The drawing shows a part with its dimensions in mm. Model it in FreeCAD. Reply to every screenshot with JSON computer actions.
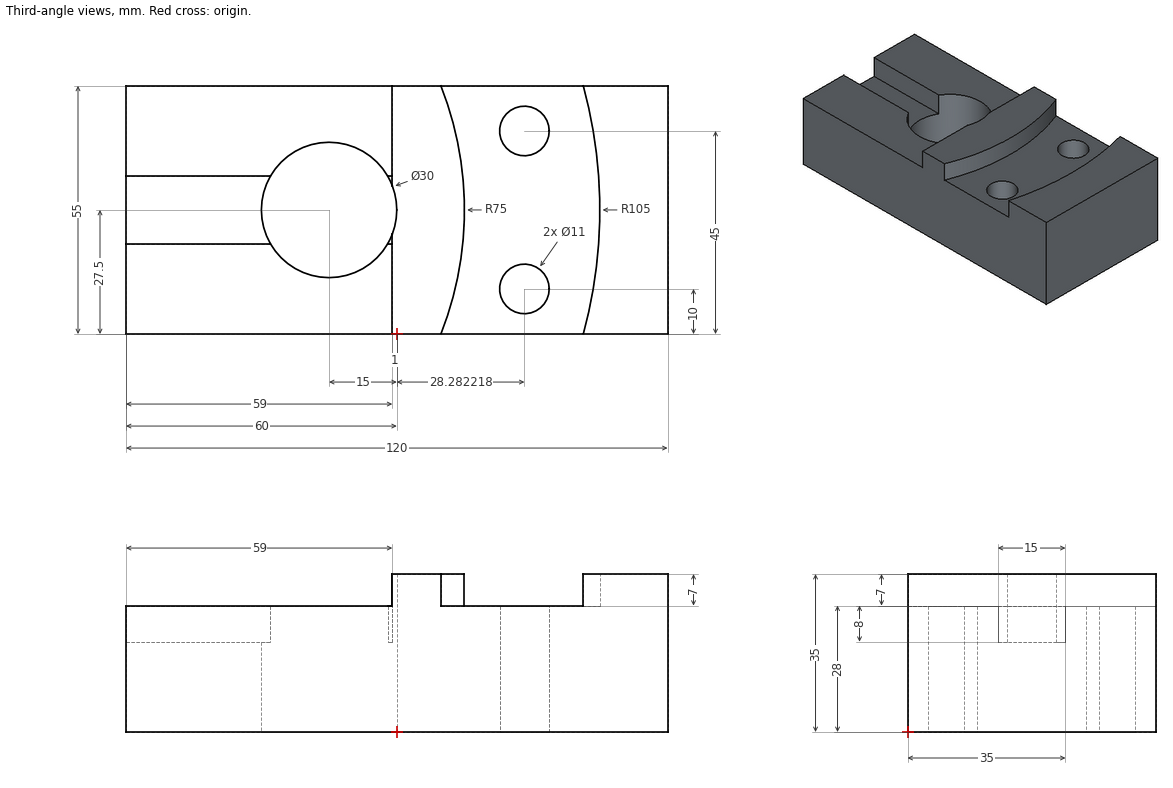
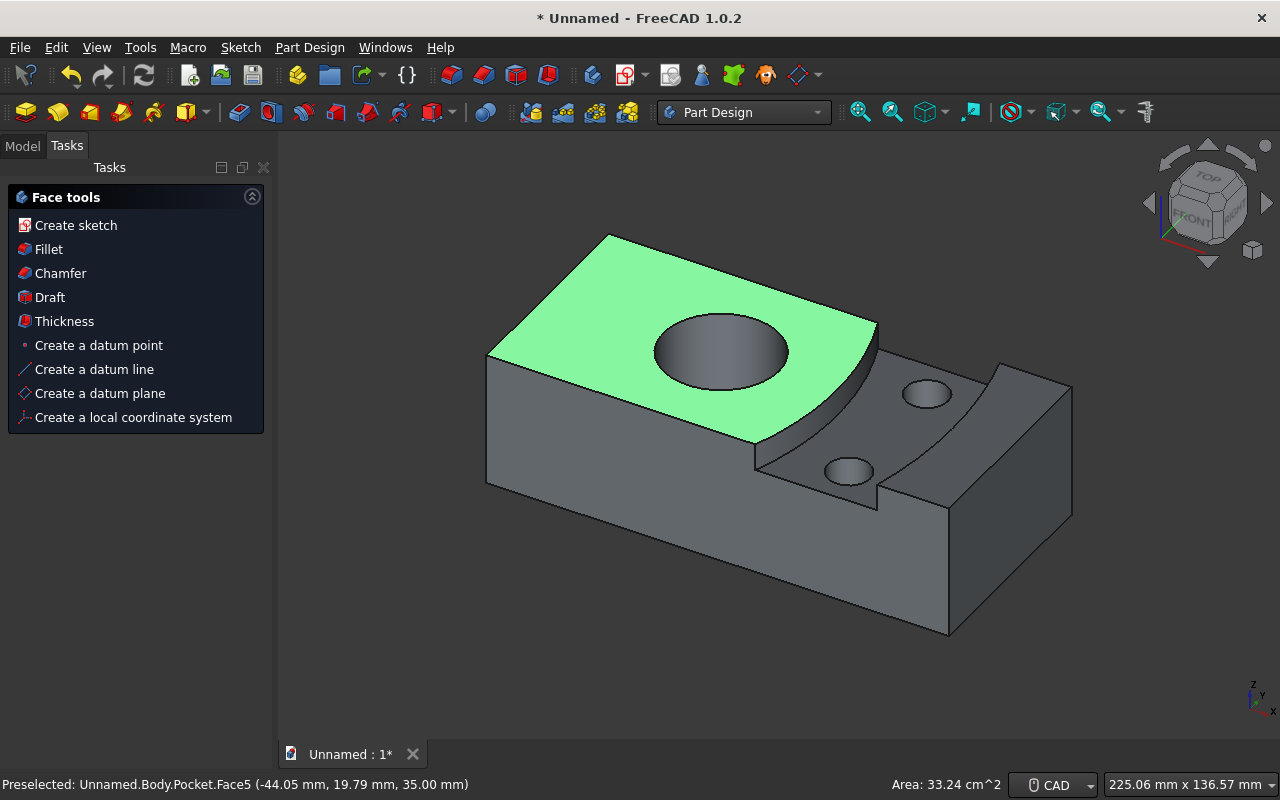
{"action": "left_click", "coordinate": [626, 76]}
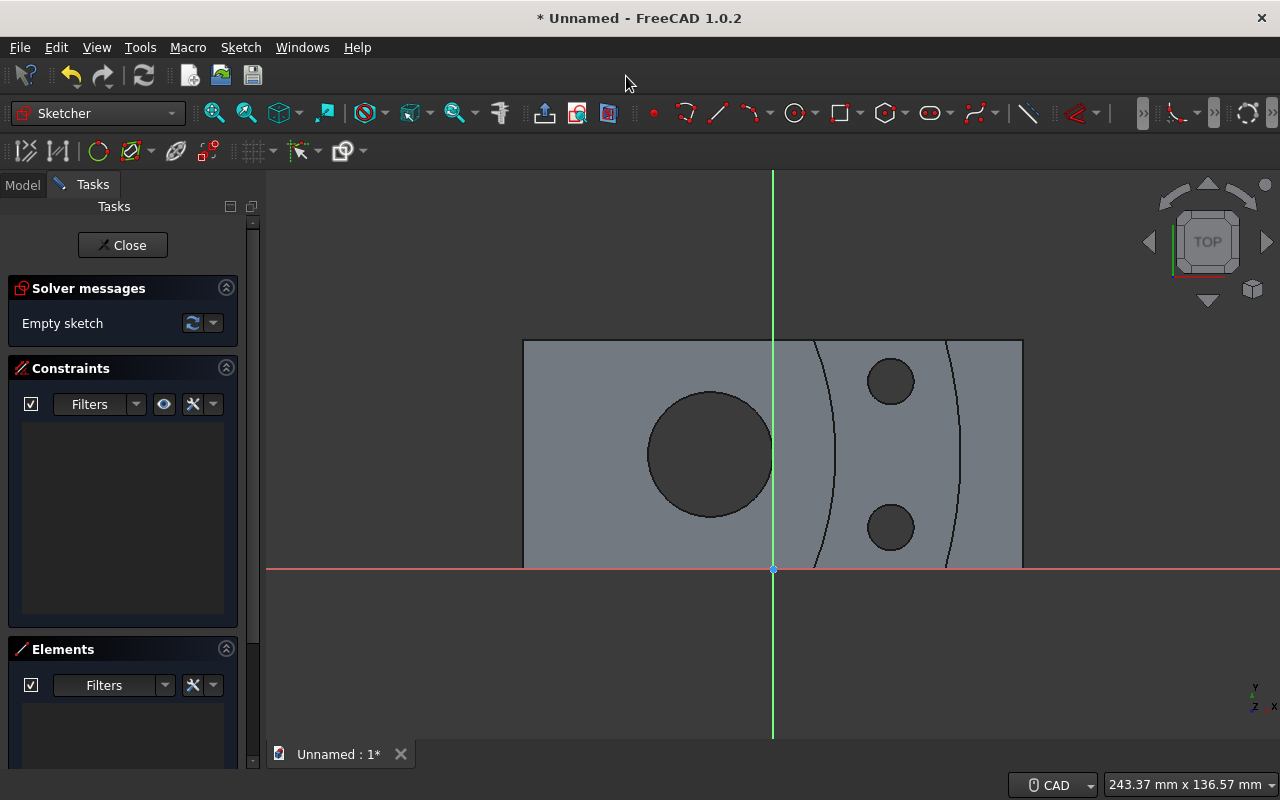
{"action": "scroll", "coordinate": [533, 455], "scroll_direction": "up", "scroll_amount": 2}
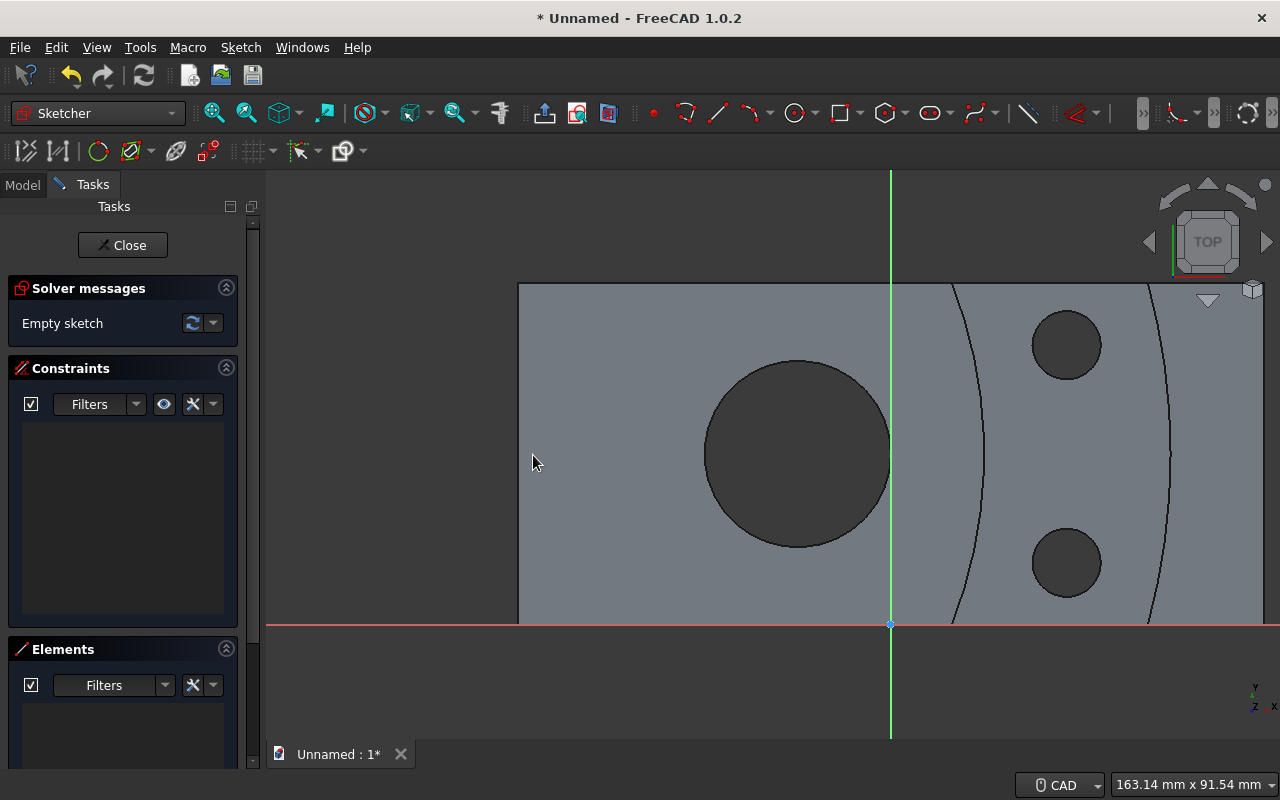
{"action": "left_click", "coordinate": [840, 114]}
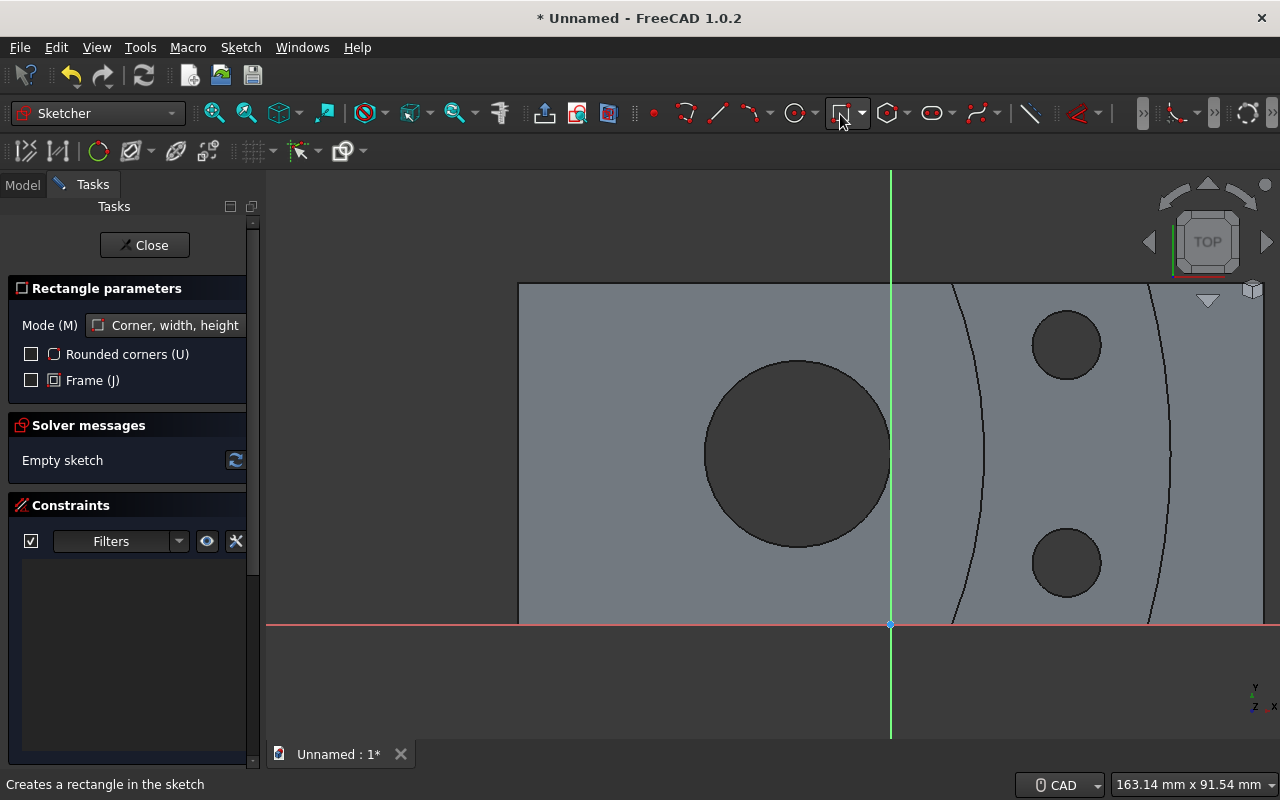
{"action": "left_click", "coordinate": [518, 283]}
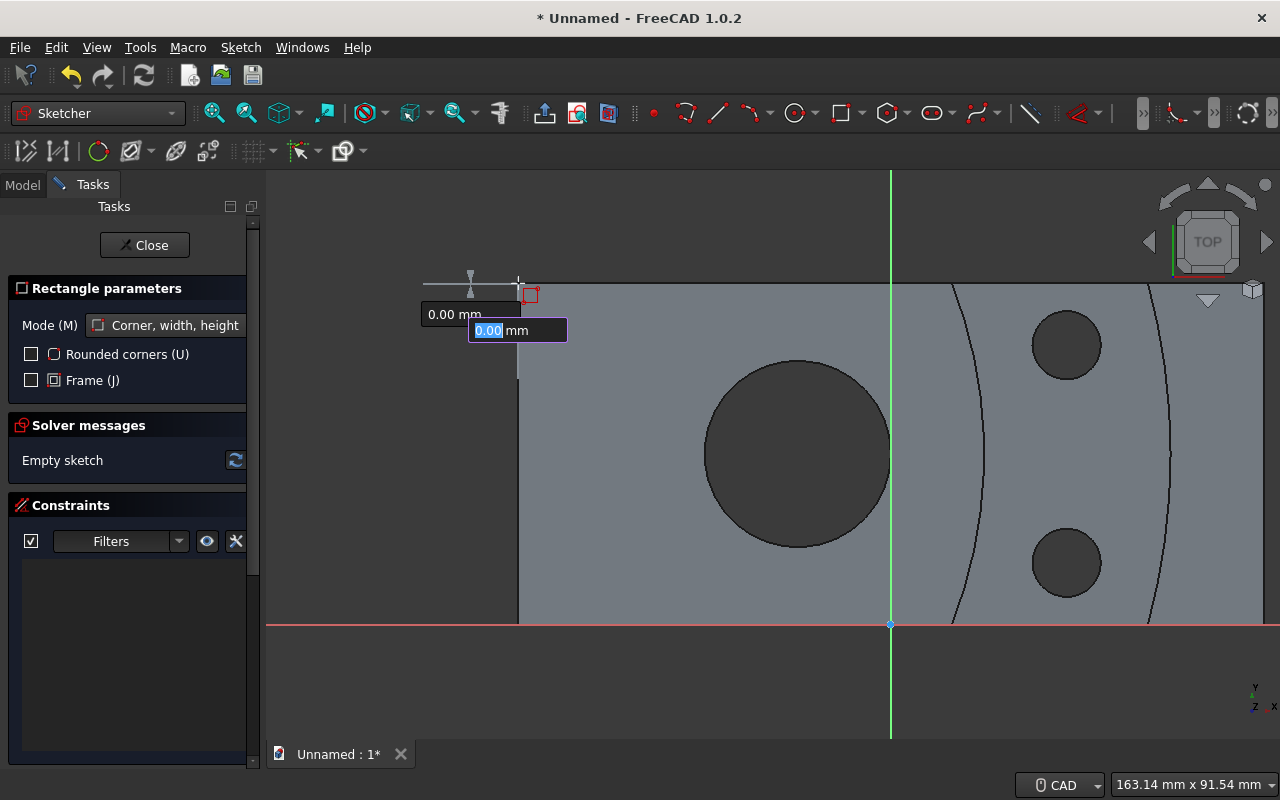
{"action": "scroll", "coordinate": [885, 625], "scroll_direction": "up", "scroll_amount": 5}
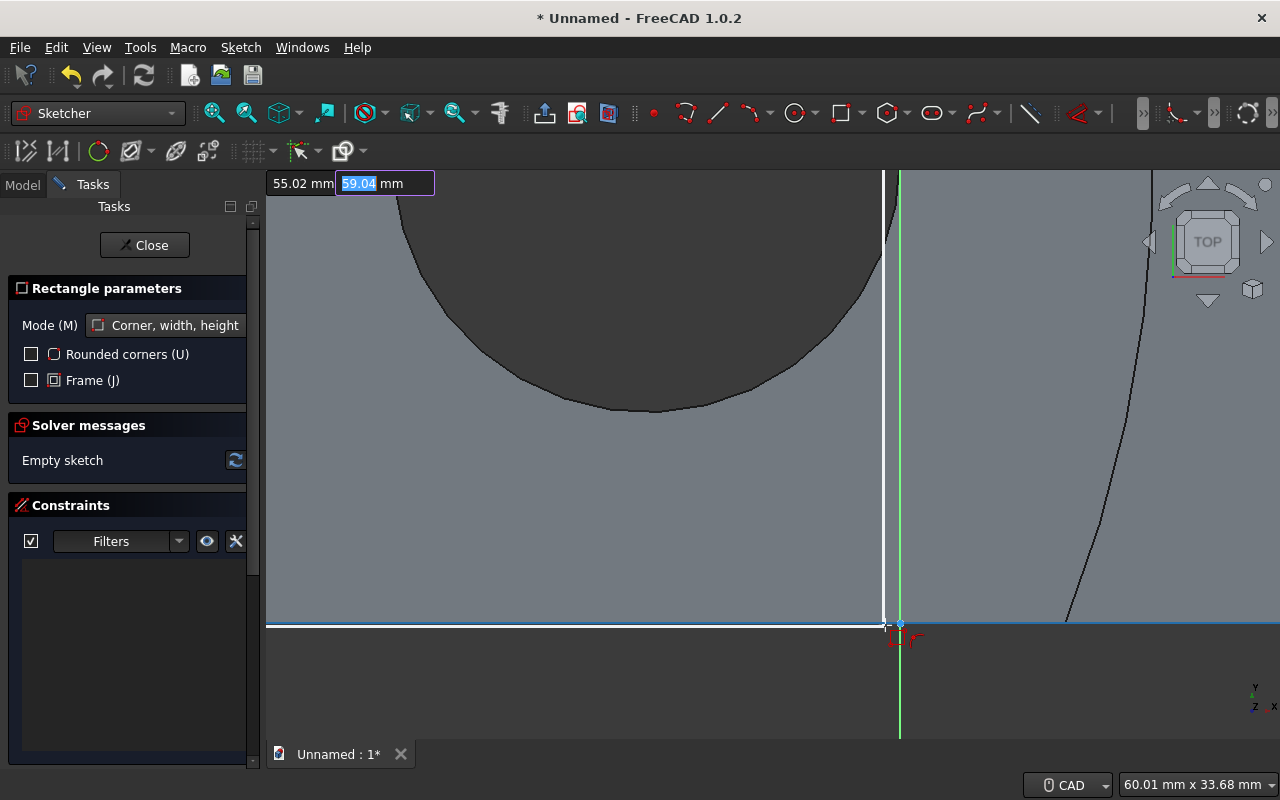
{"action": "left_click", "coordinate": [883, 623]}
{"action": "key", "text": "Escape"}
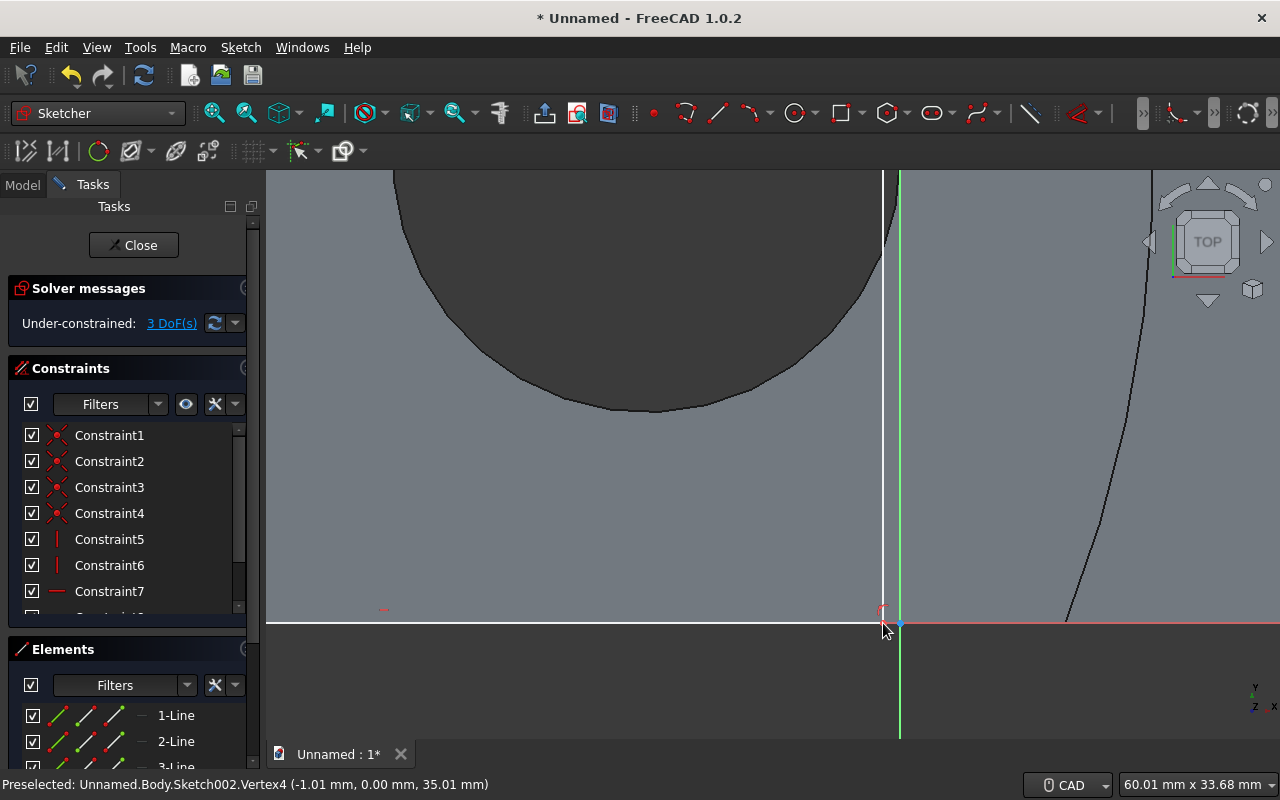
{"action": "key", "text": "d"}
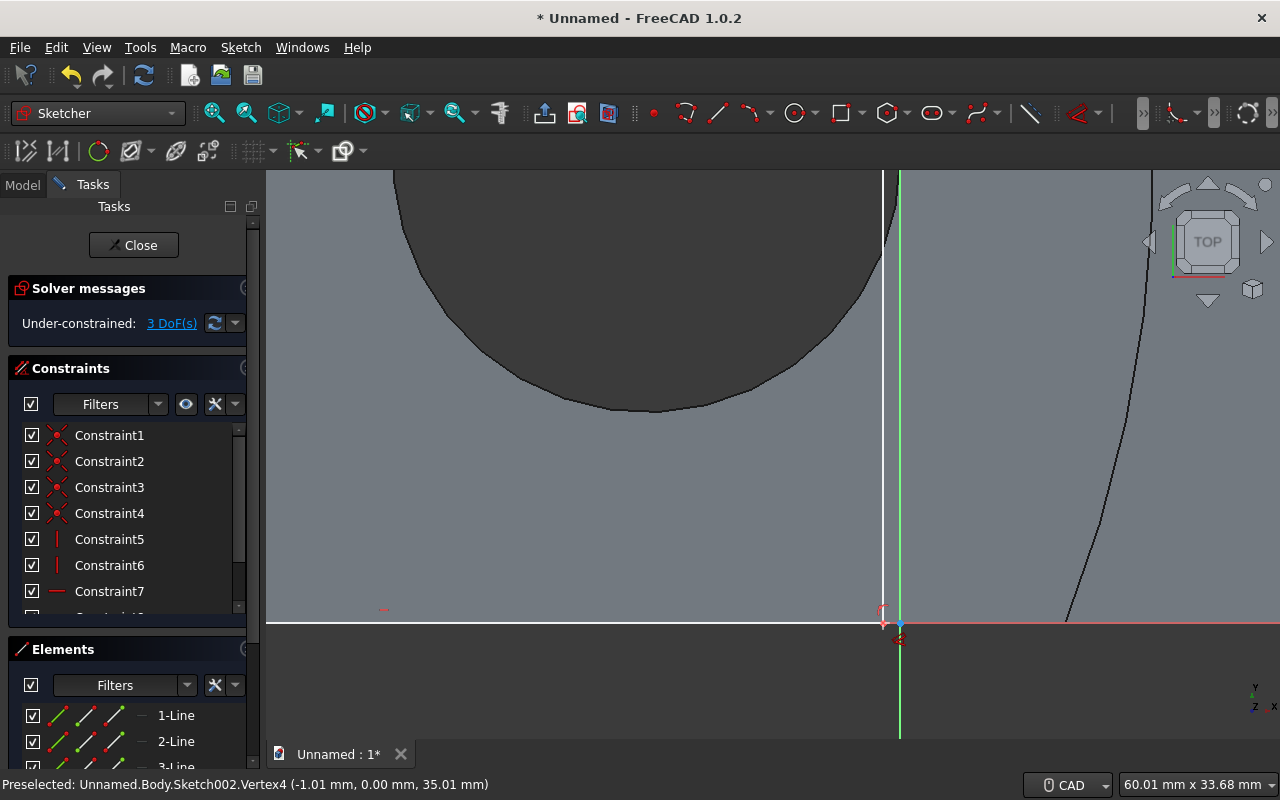
{"action": "scroll", "coordinate": [886, 627], "scroll_direction": "down", "scroll_amount": 5}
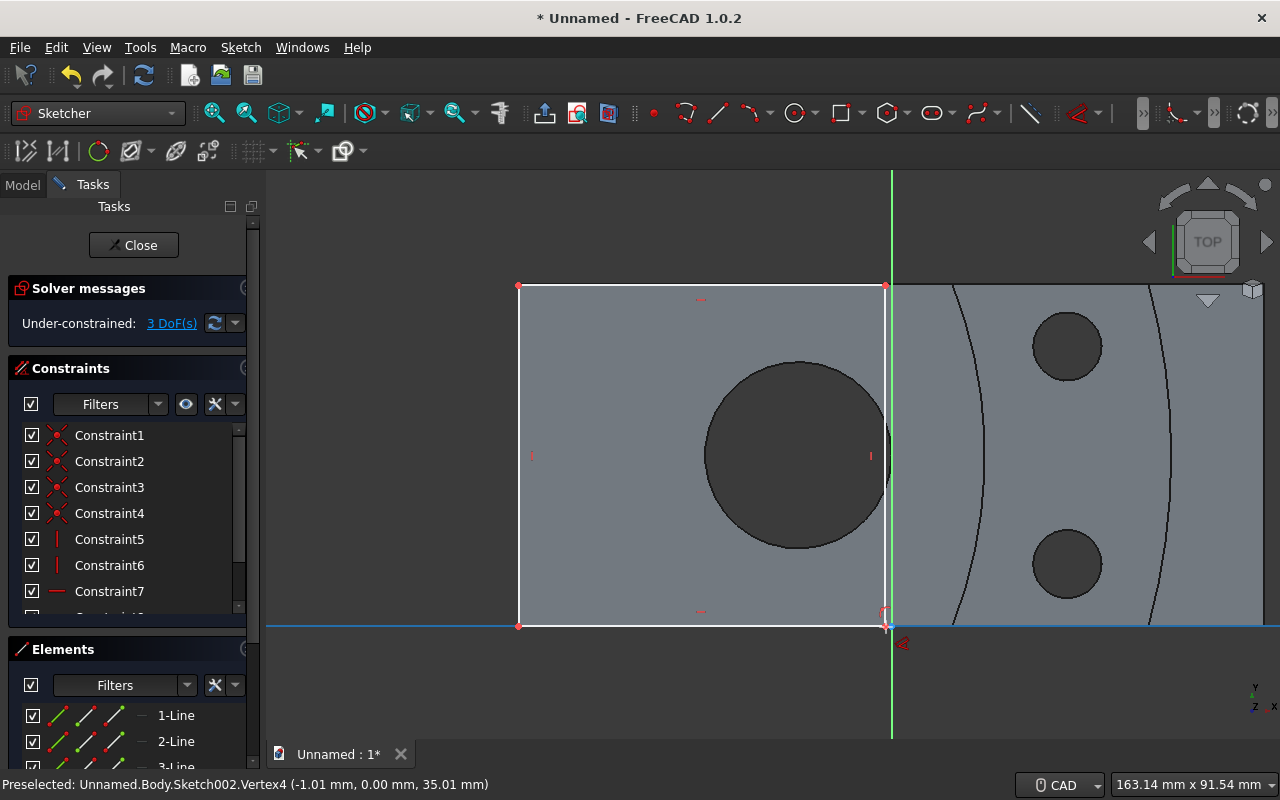
{"action": "left_click", "coordinate": [519, 388]}
{"action": "left_click", "coordinate": [485, 456]}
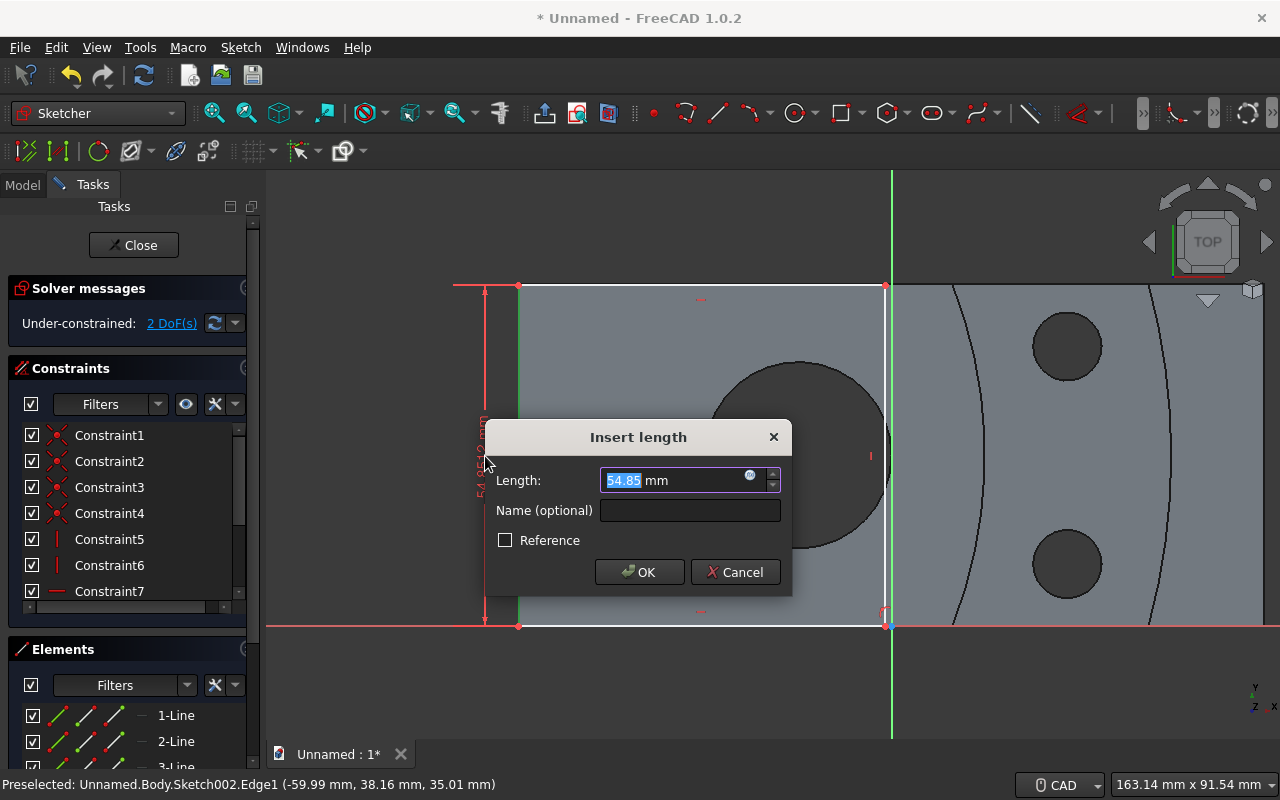
{"action": "type", "text": "55"}
{"action": "key", "text": "Return"}